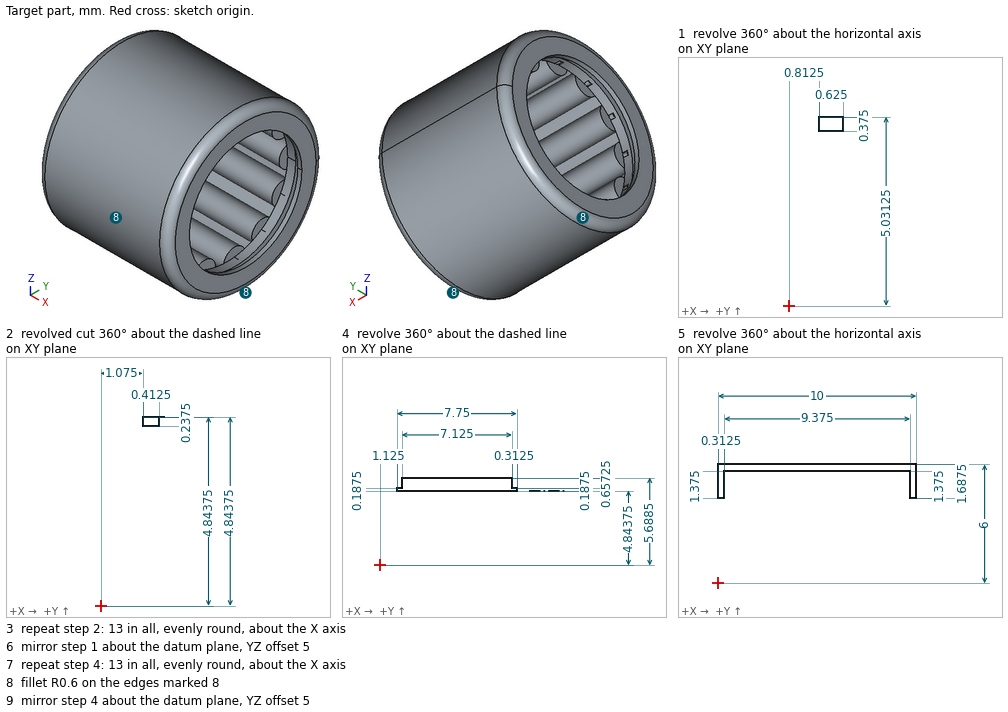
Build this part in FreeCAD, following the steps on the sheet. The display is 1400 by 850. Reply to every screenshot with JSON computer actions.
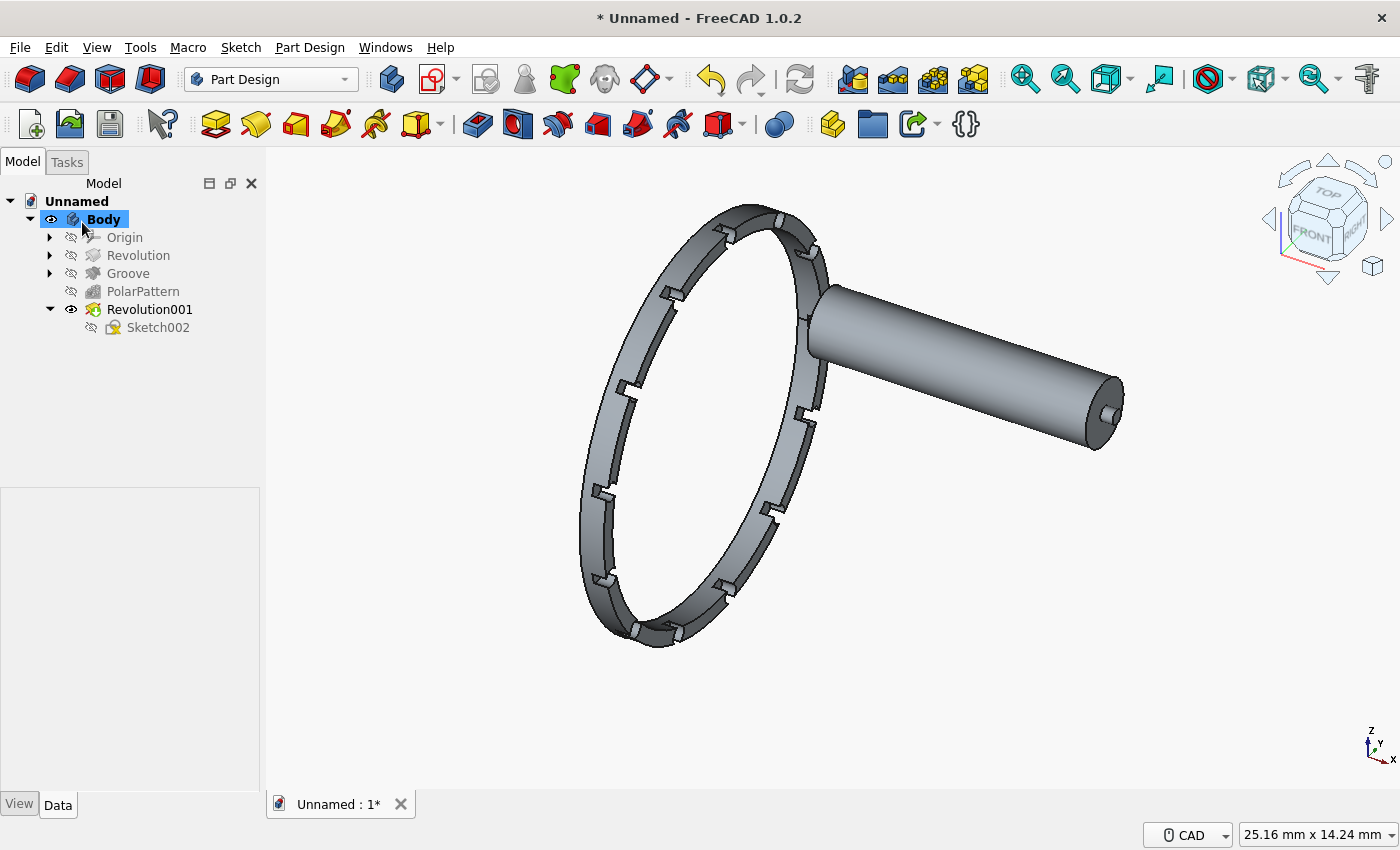
{"action": "key", "text": "v f"}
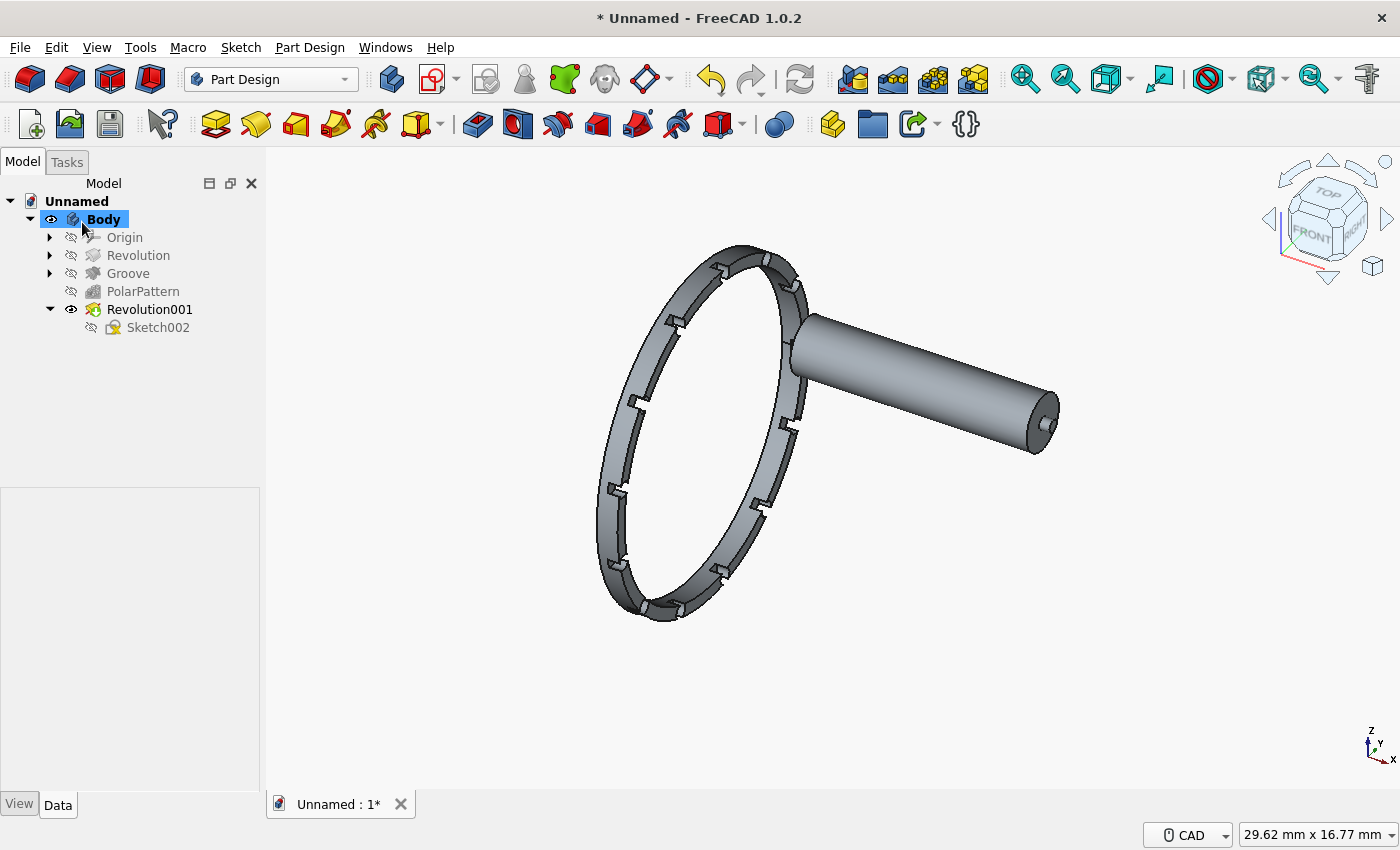
{"action": "left_click", "coordinate": [432, 80]}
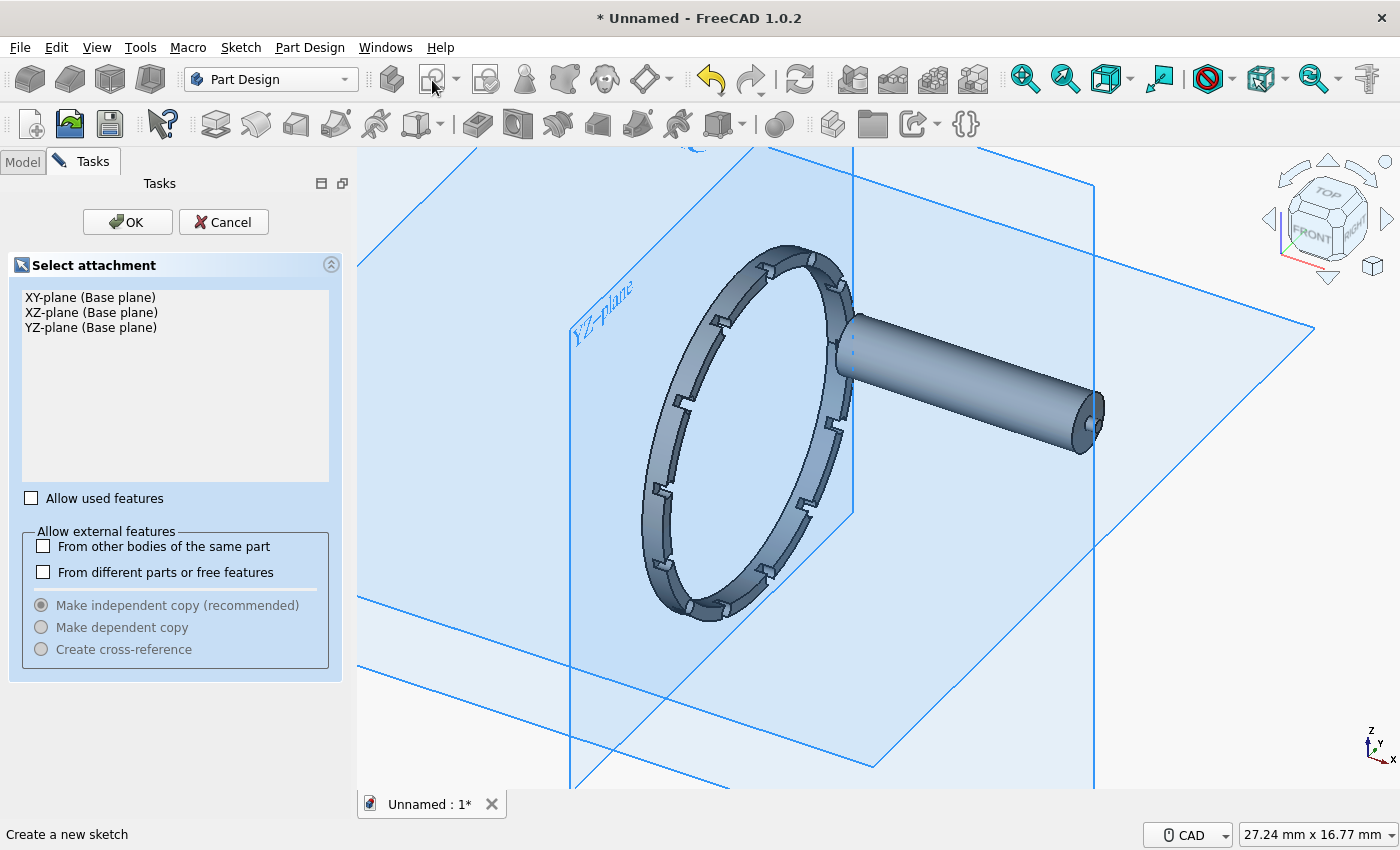
{"action": "left_click", "coordinate": [82, 298]}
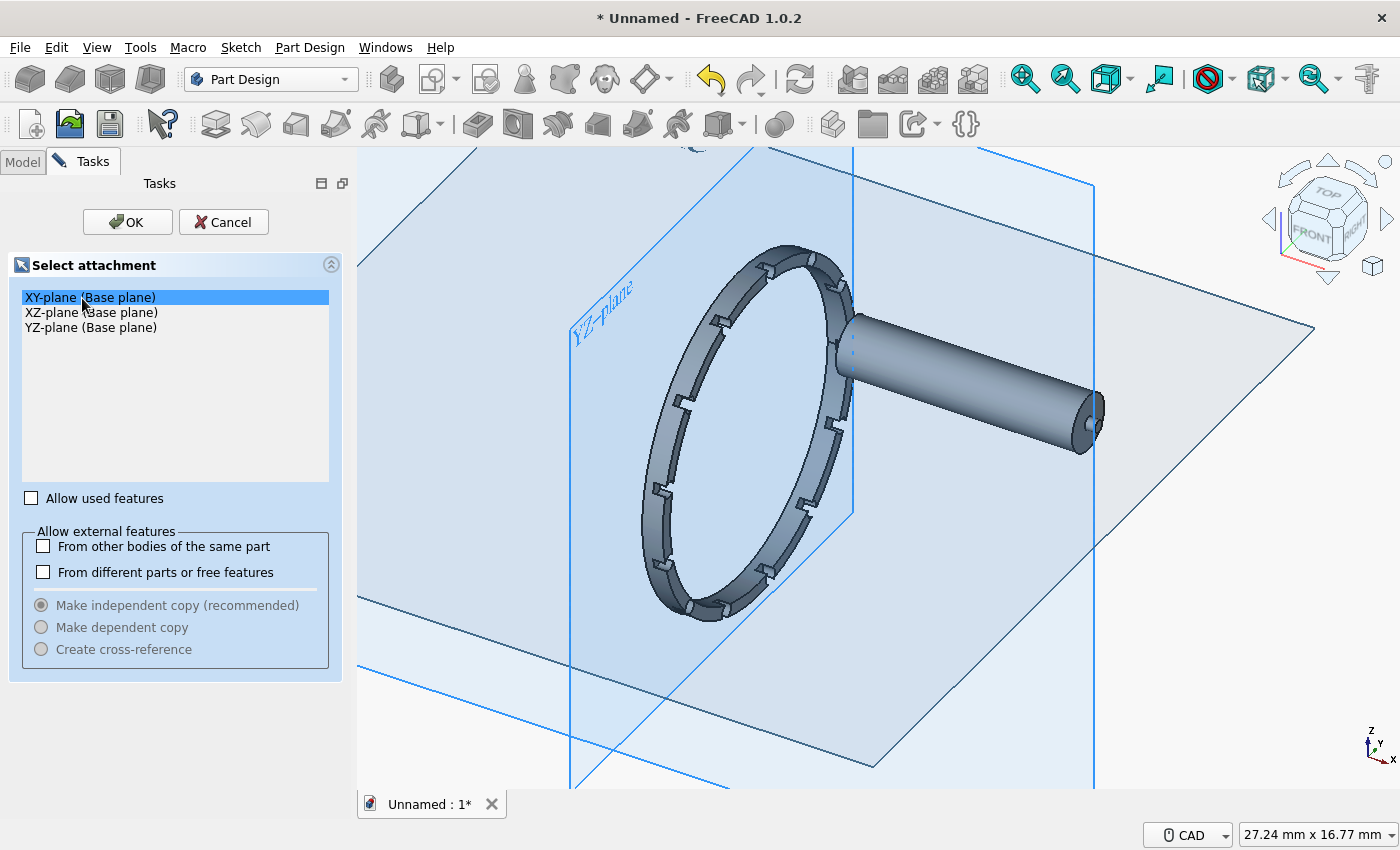
{"action": "left_click", "coordinate": [128, 222]}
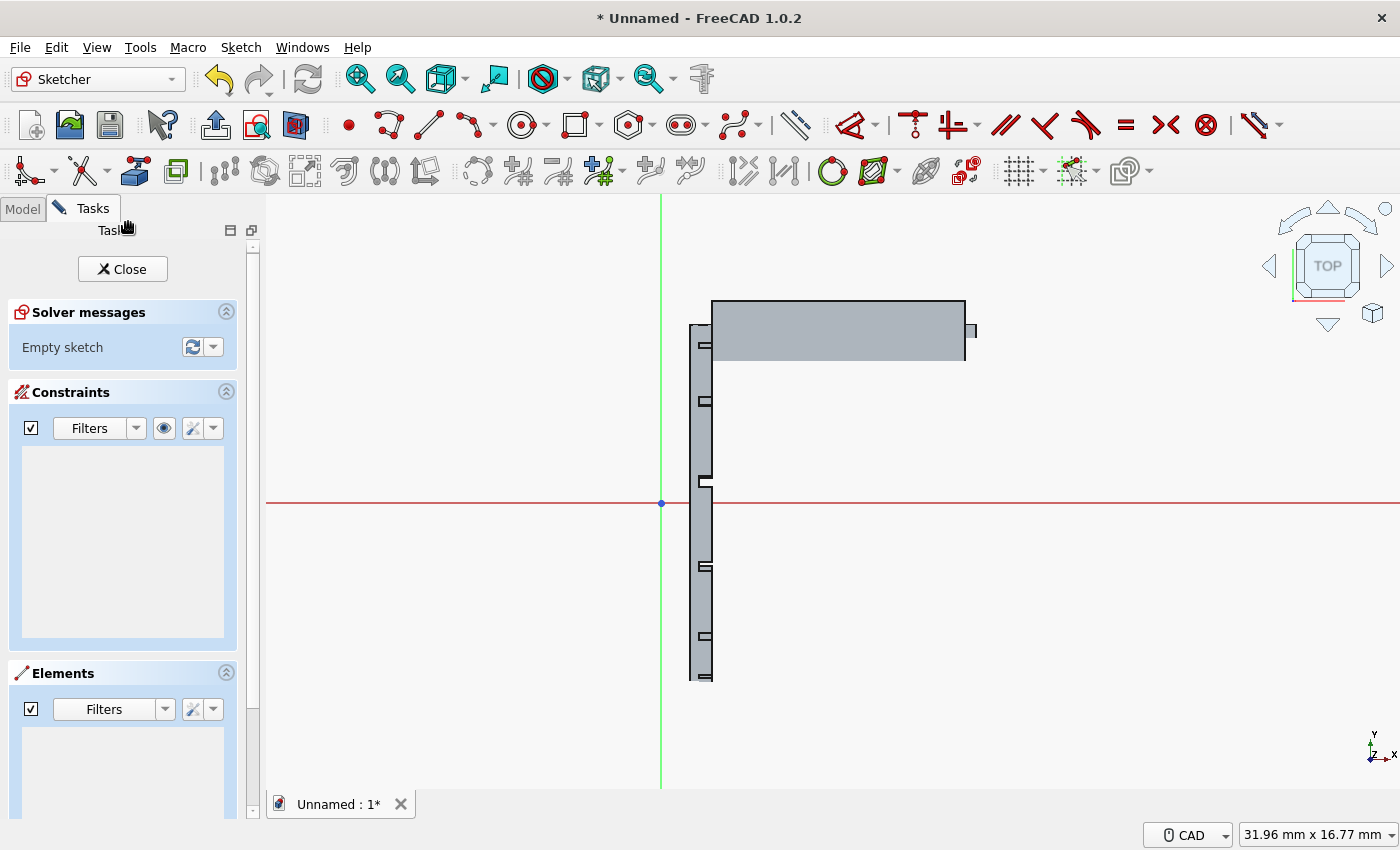
{"action": "key", "text": "q s"}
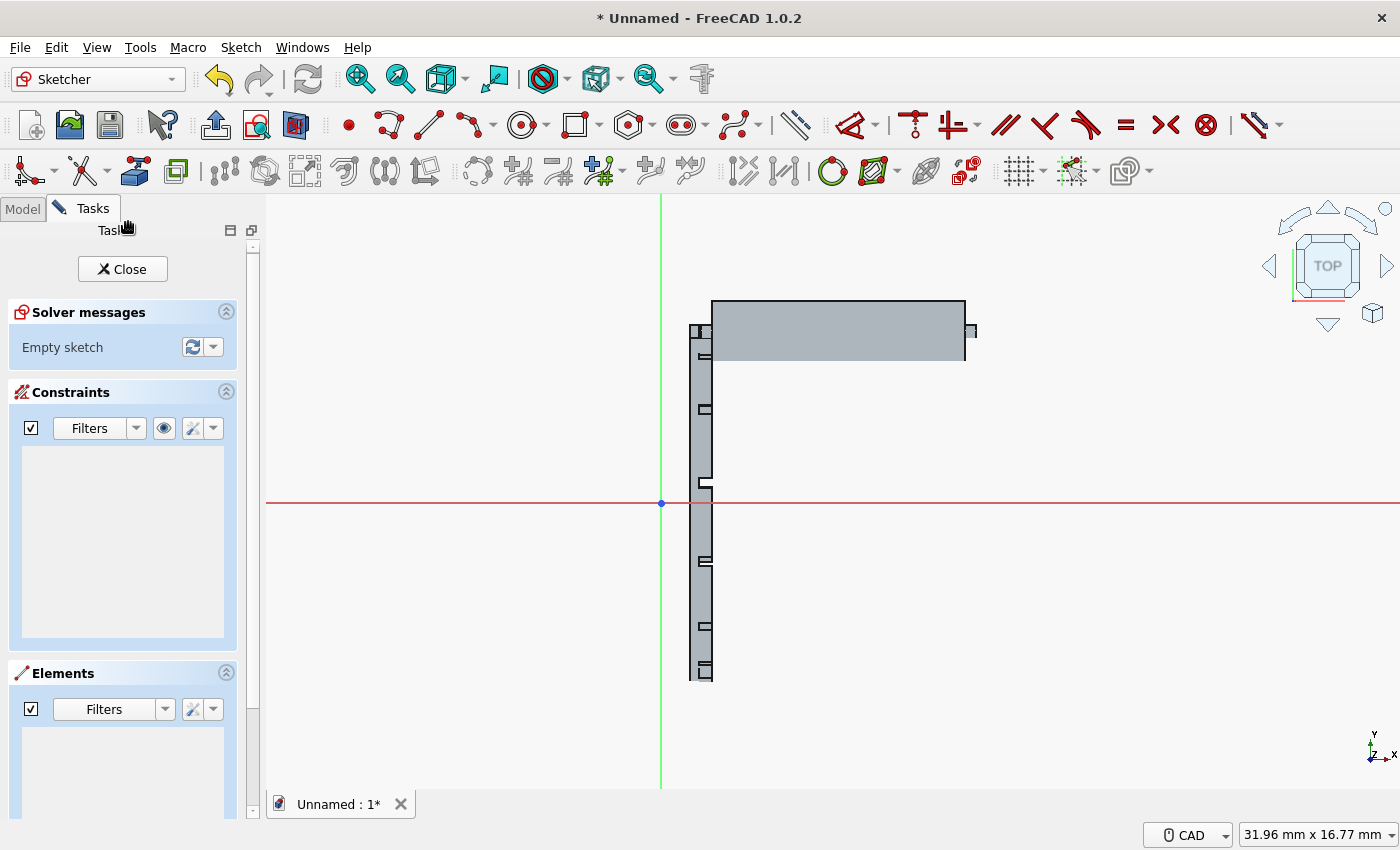
{"action": "scroll", "coordinate": [929, 281], "scroll_direction": "up", "scroll_amount": 3}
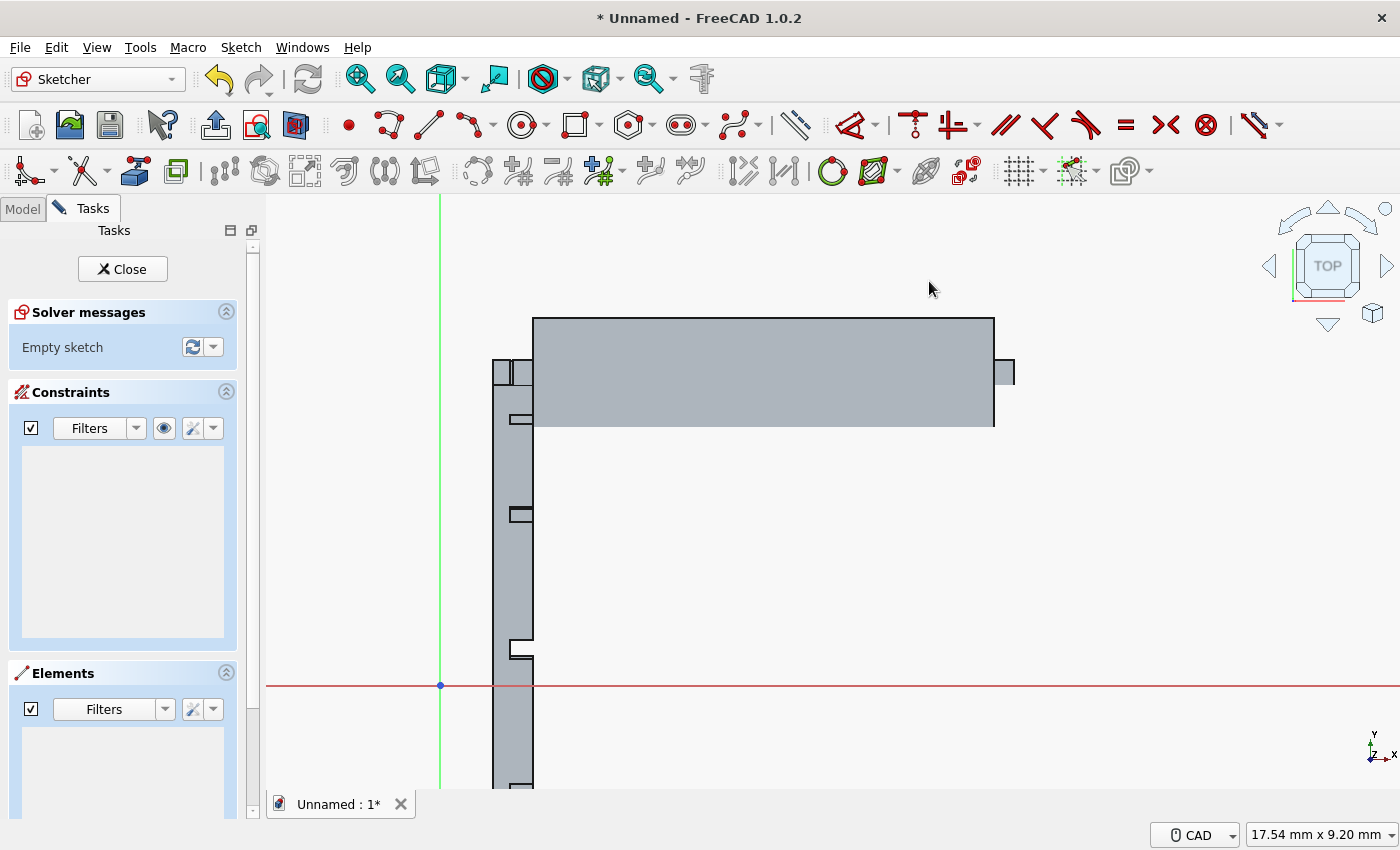
{"action": "key", "text": "g m"}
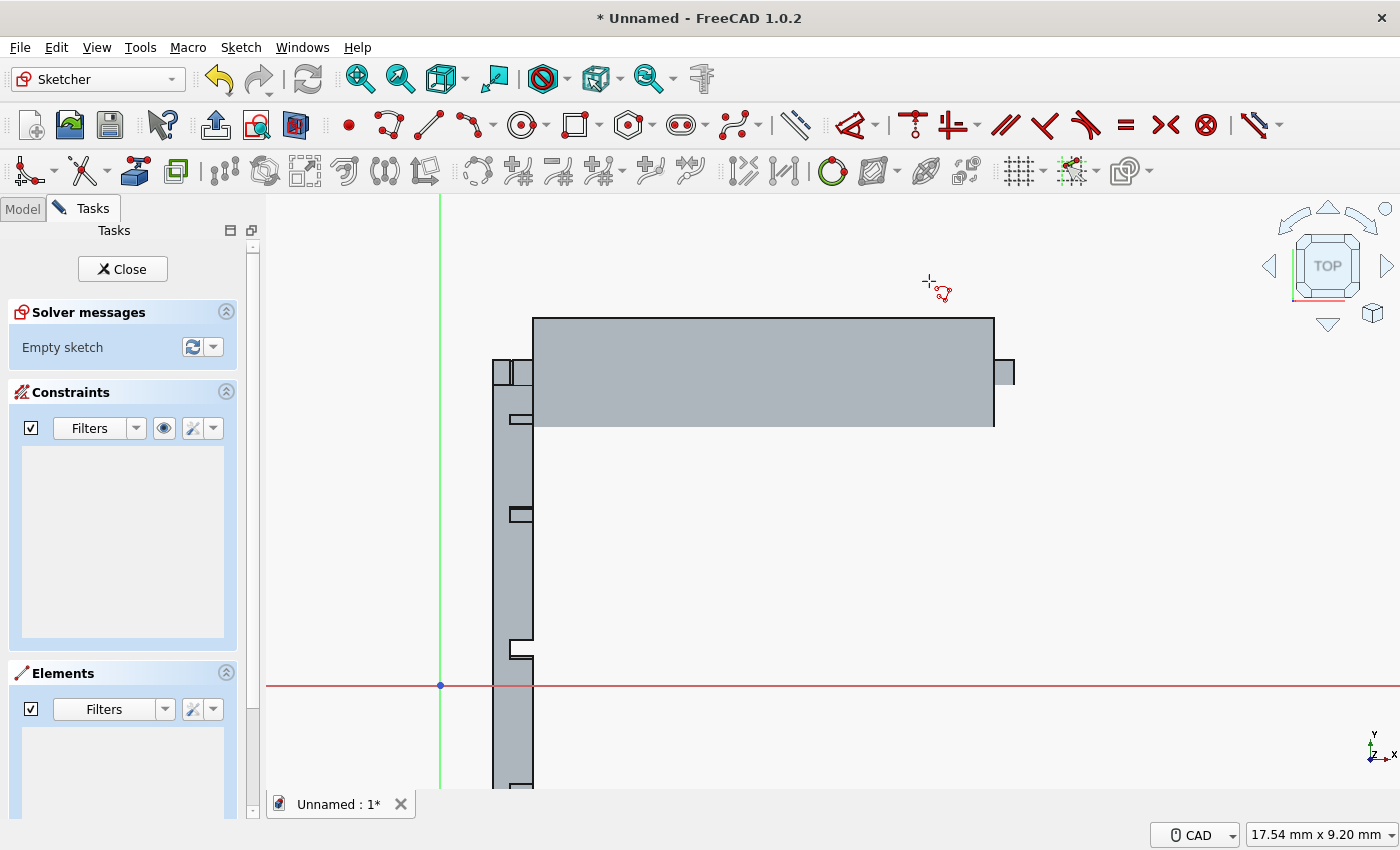
{"action": "left_click", "coordinate": [440, 407]}
{"action": "left_click", "coordinate": [461, 407]}
{"action": "left_click", "coordinate": [461, 318]}
{"action": "left_click", "coordinate": [1067, 318]}
{"action": "left_click", "coordinate": [1067, 407]}
{"action": "left_click", "coordinate": [1087, 407]}
{"action": "left_click", "coordinate": [1087, 298]}
{"action": "left_click", "coordinate": [449, 298]}